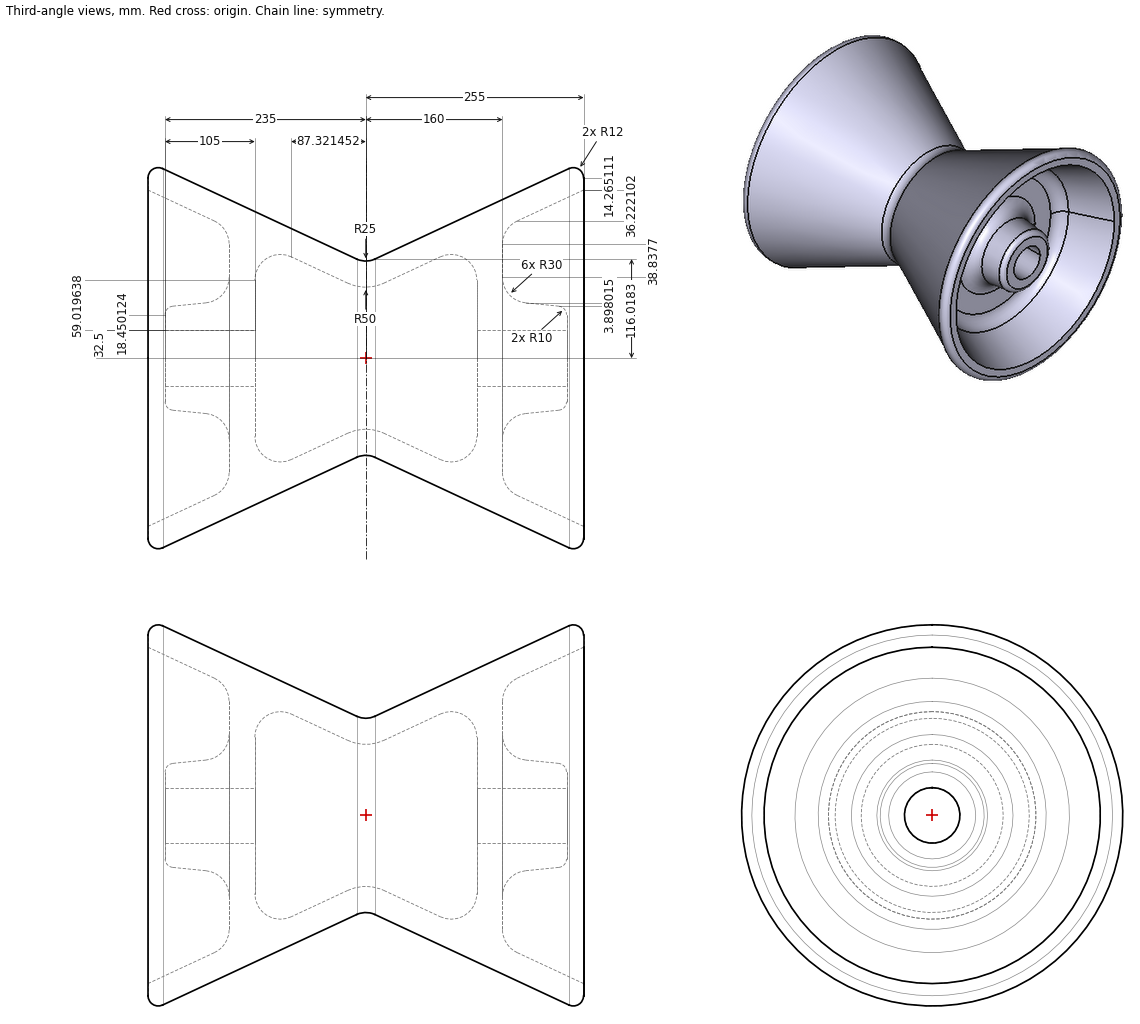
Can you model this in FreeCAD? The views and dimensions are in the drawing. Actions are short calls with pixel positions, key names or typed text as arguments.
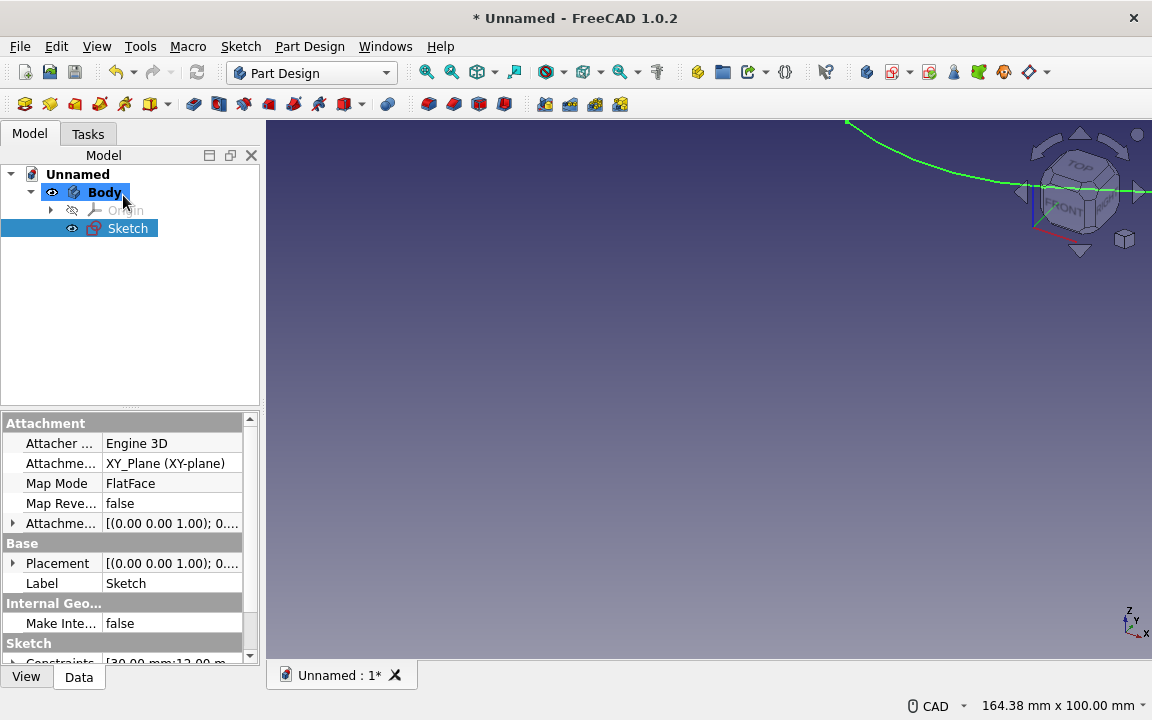
click(50, 104)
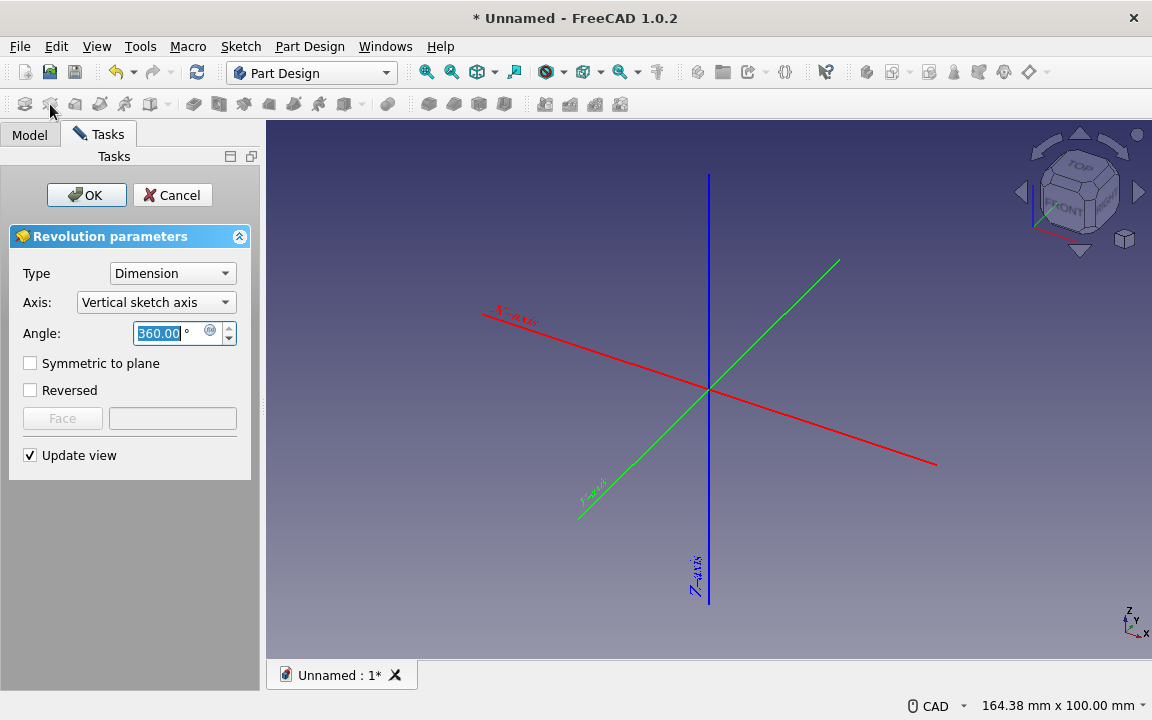
click(157, 302)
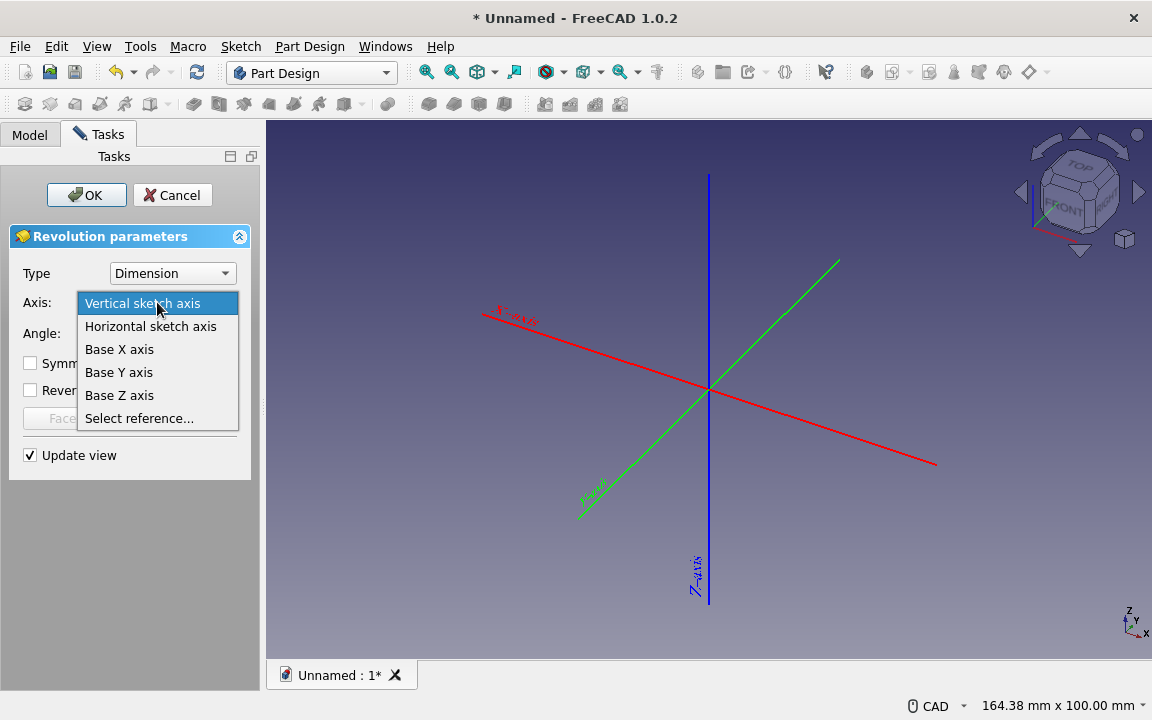
click(156, 326)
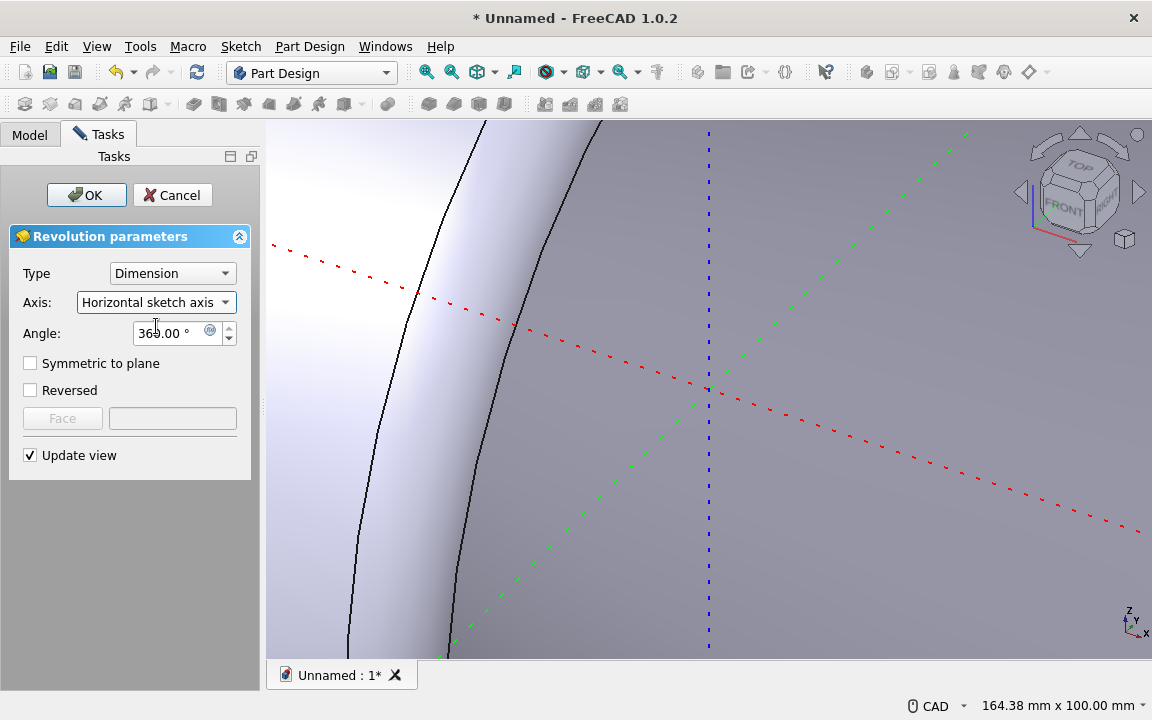
click(87, 195)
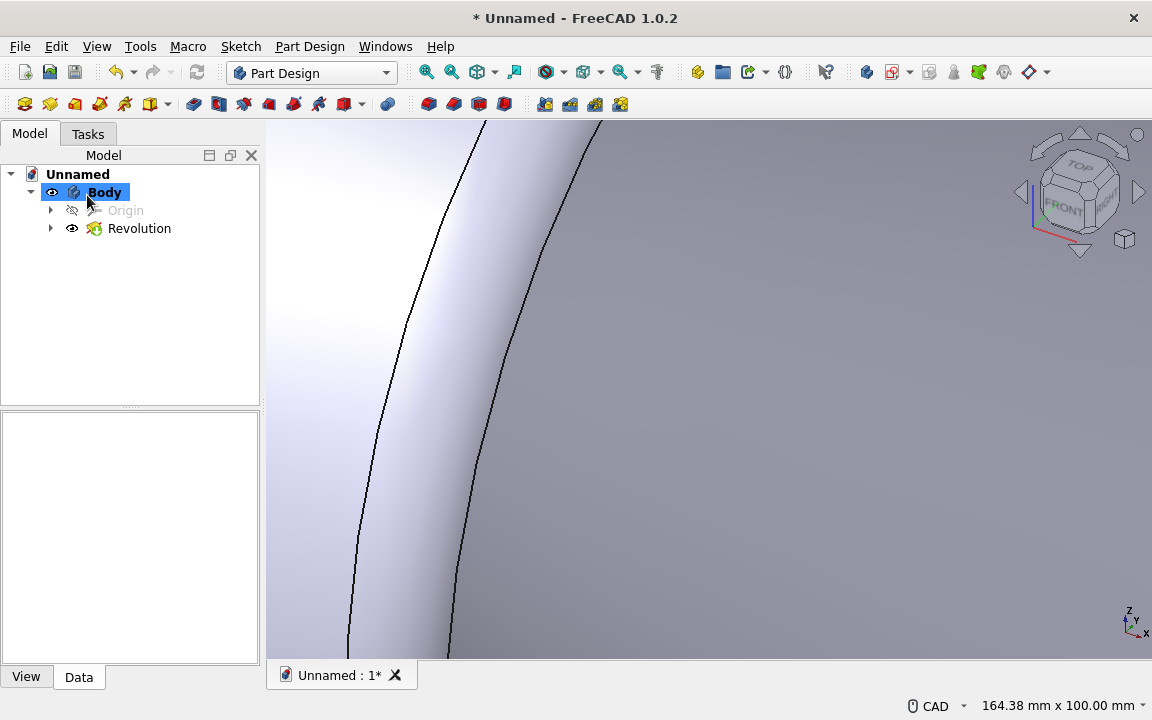
key(0)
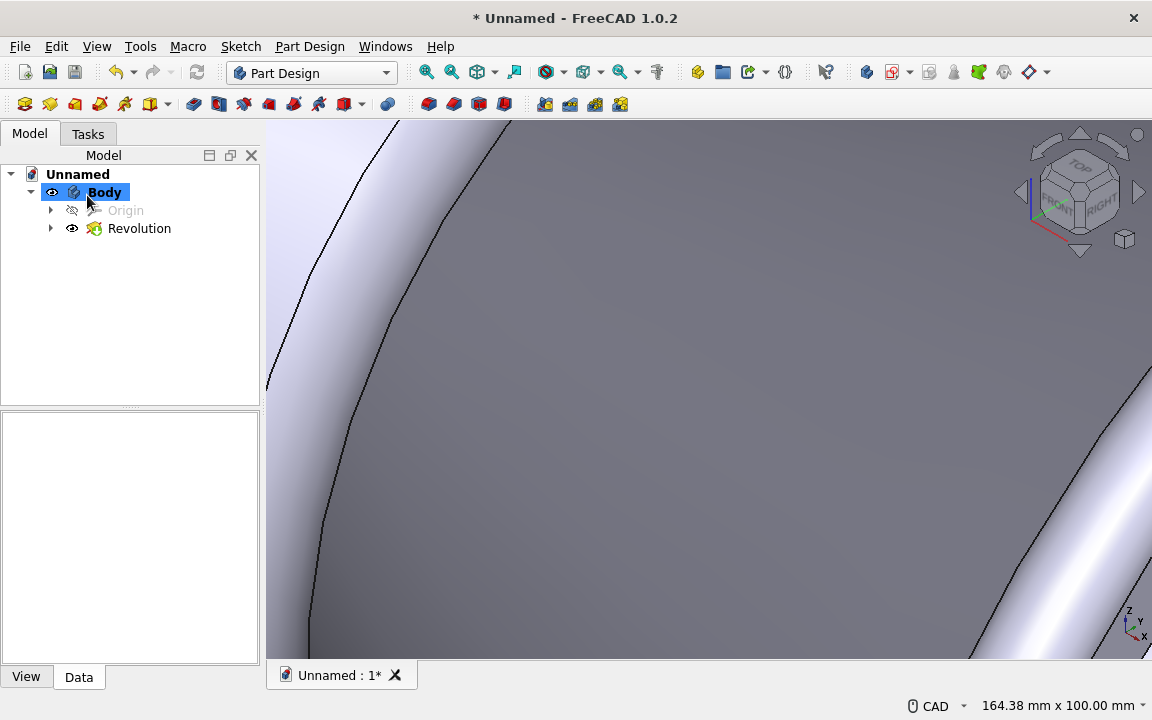
click(427, 72)